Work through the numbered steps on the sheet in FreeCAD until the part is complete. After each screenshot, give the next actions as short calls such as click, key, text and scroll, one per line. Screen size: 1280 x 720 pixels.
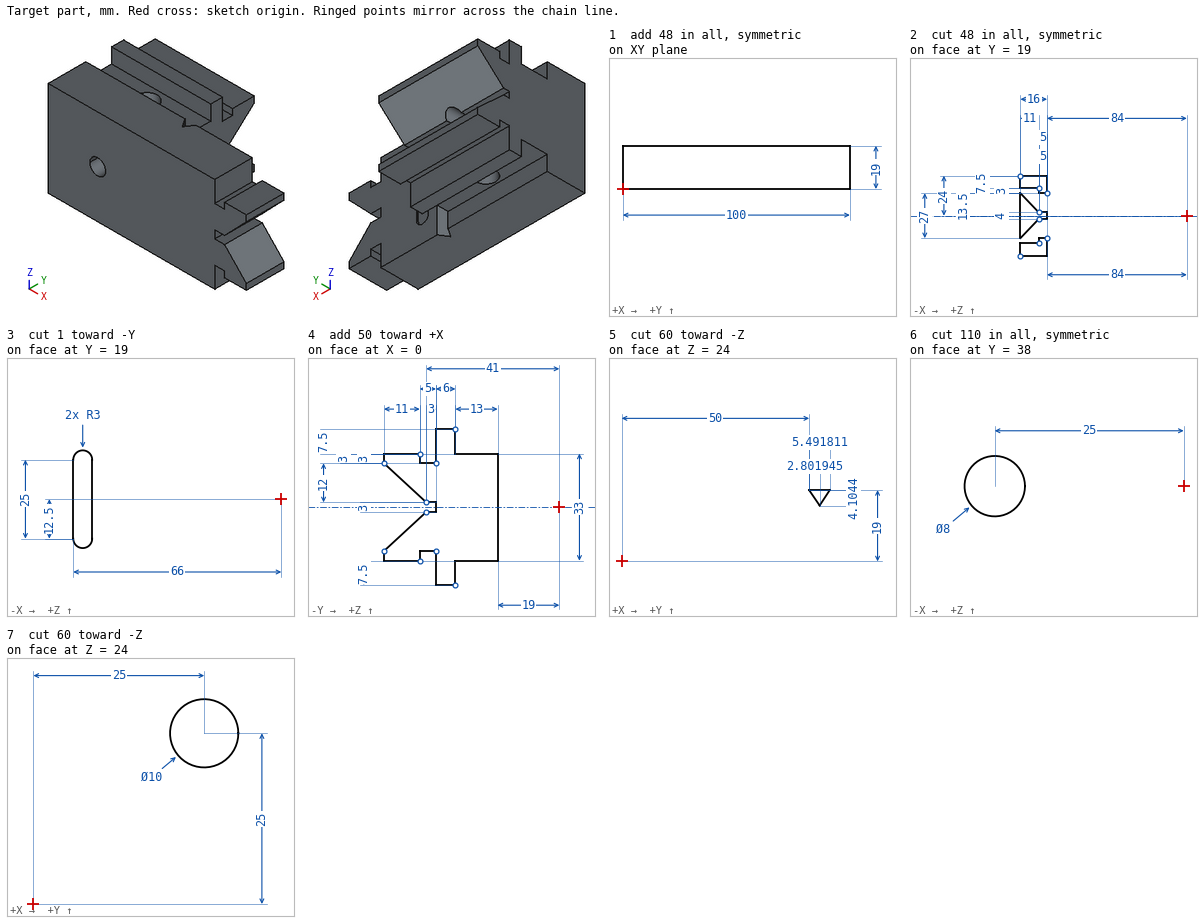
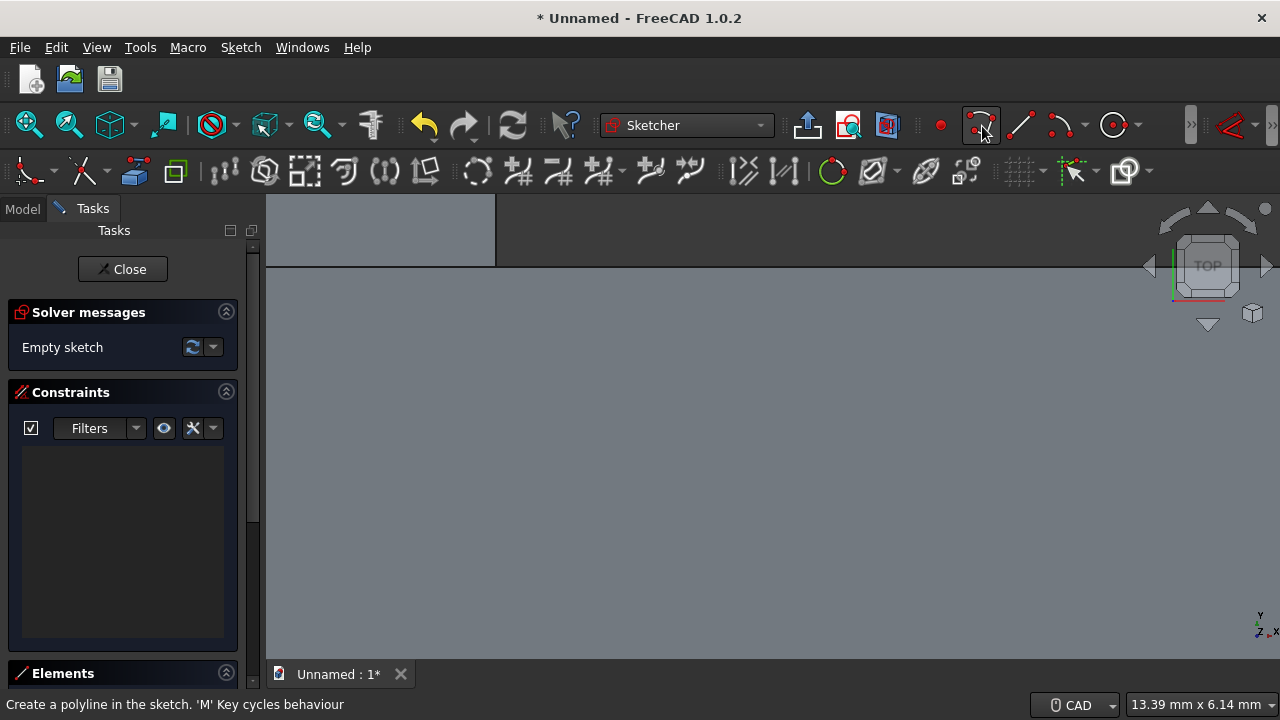
click(496, 267)
click(708, 578)
click(912, 267)
click(496, 268)
key(Escape)
key(Escape)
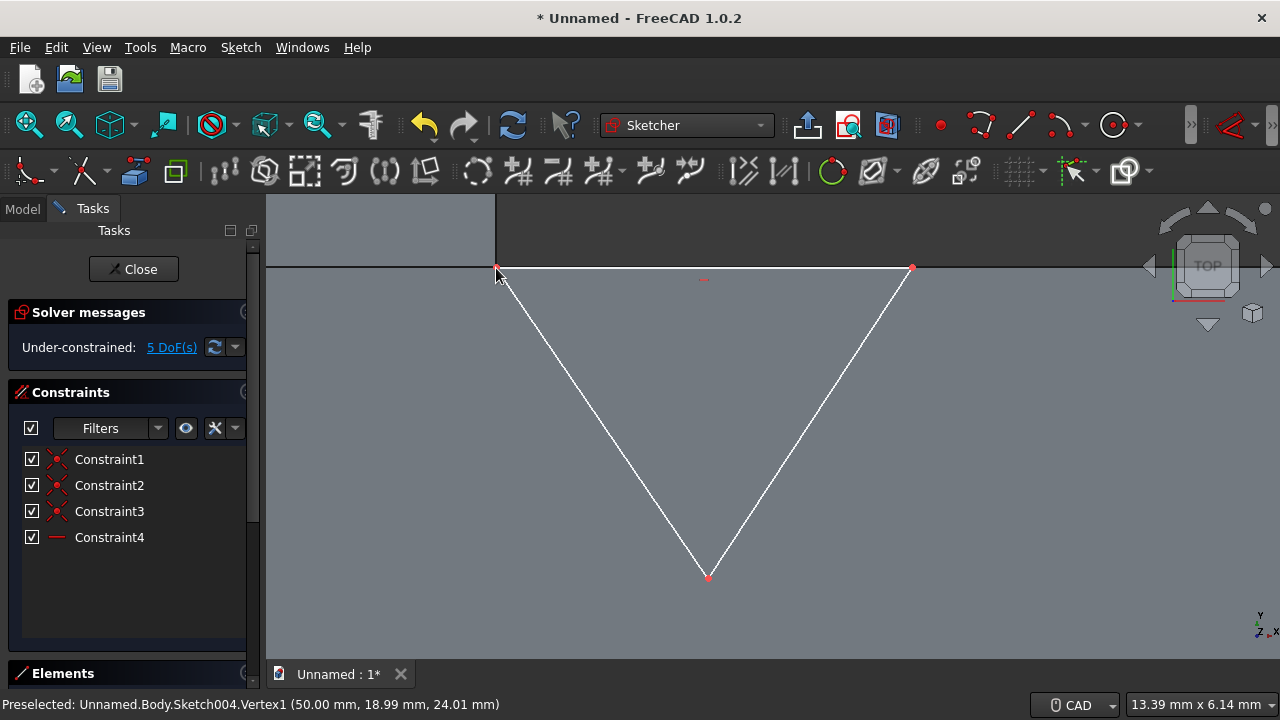
click(1230, 126)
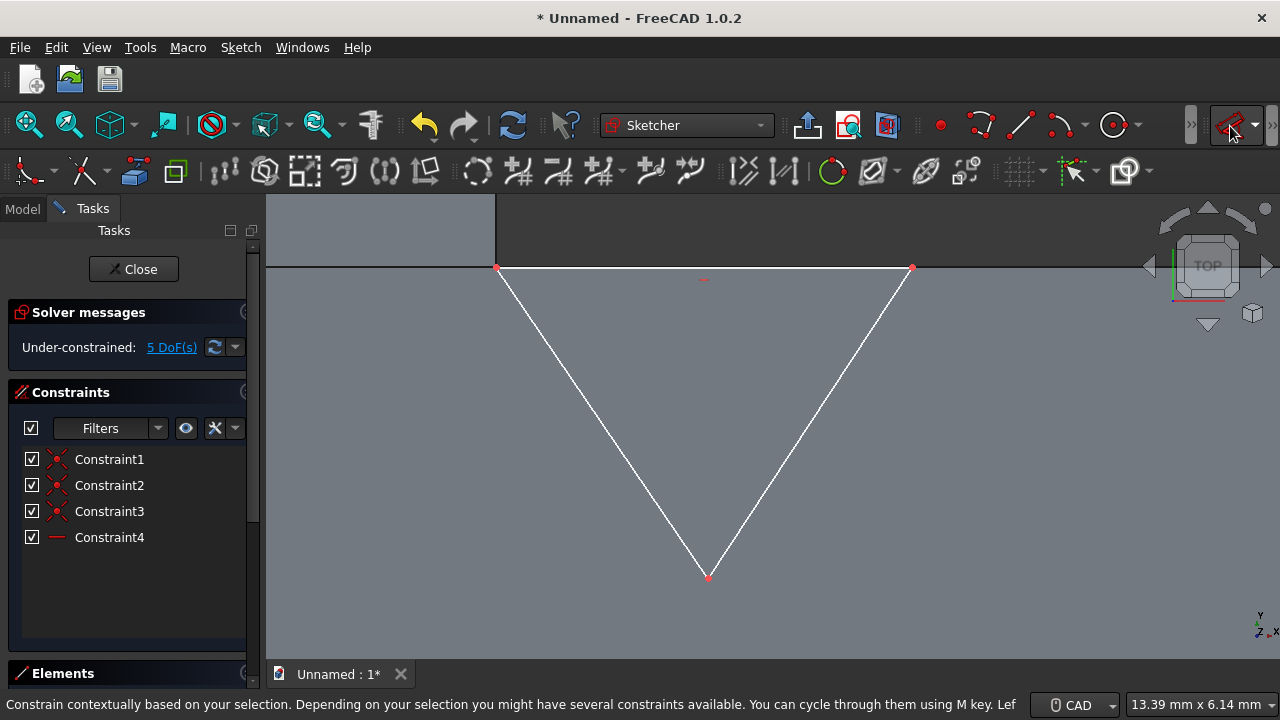
click(496, 268)
click(395, 234)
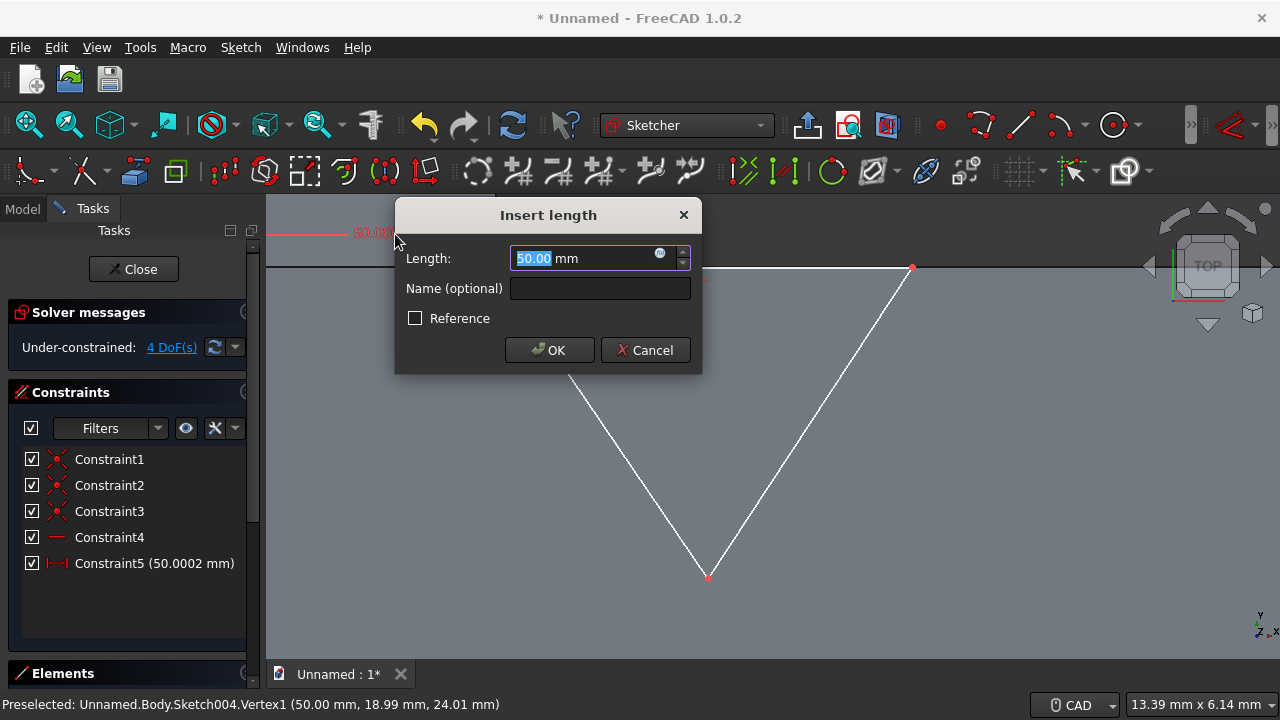
text(50)
key(Return)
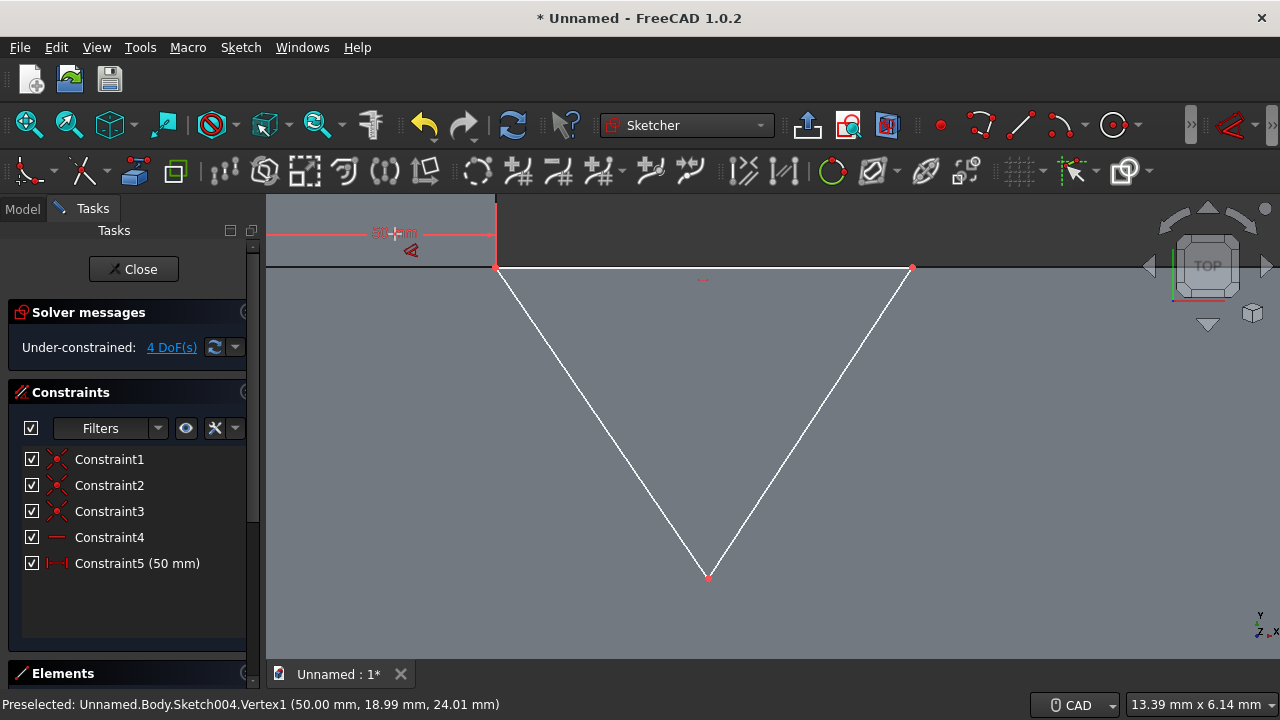
click(496, 268)
click(530, 450)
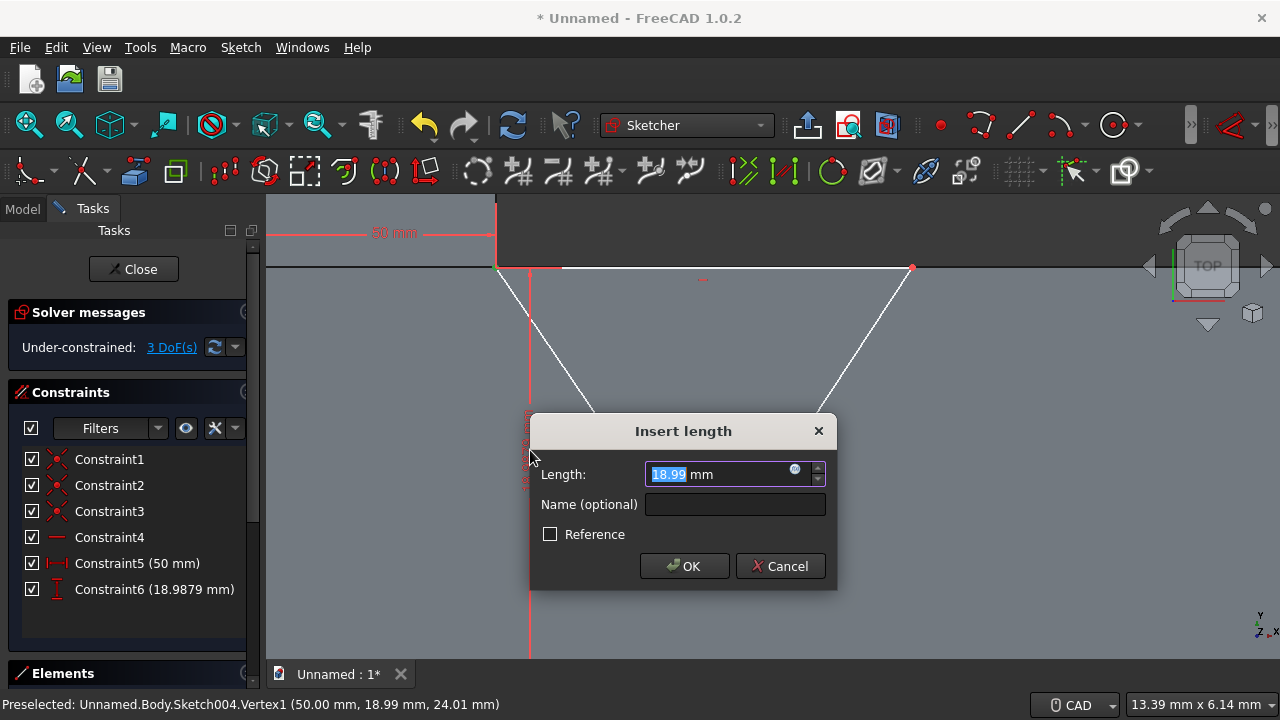
text(19)
key(Return)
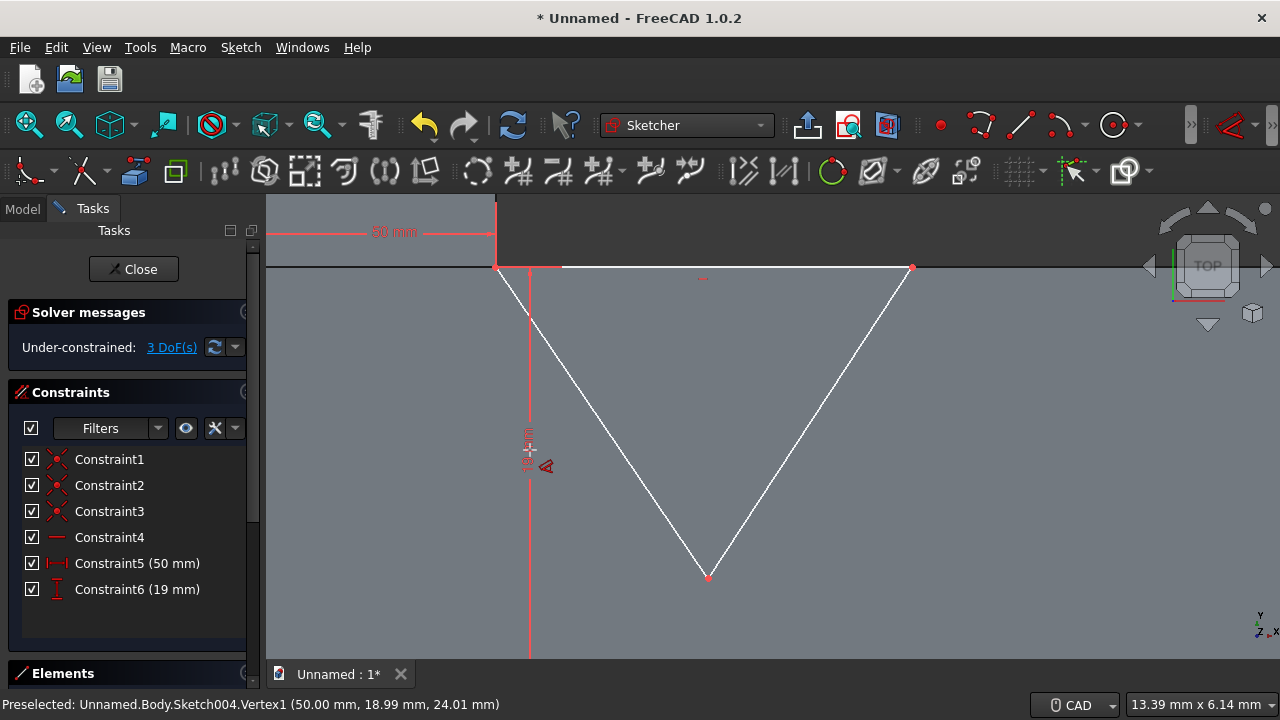
click(560, 361)
click(462, 423)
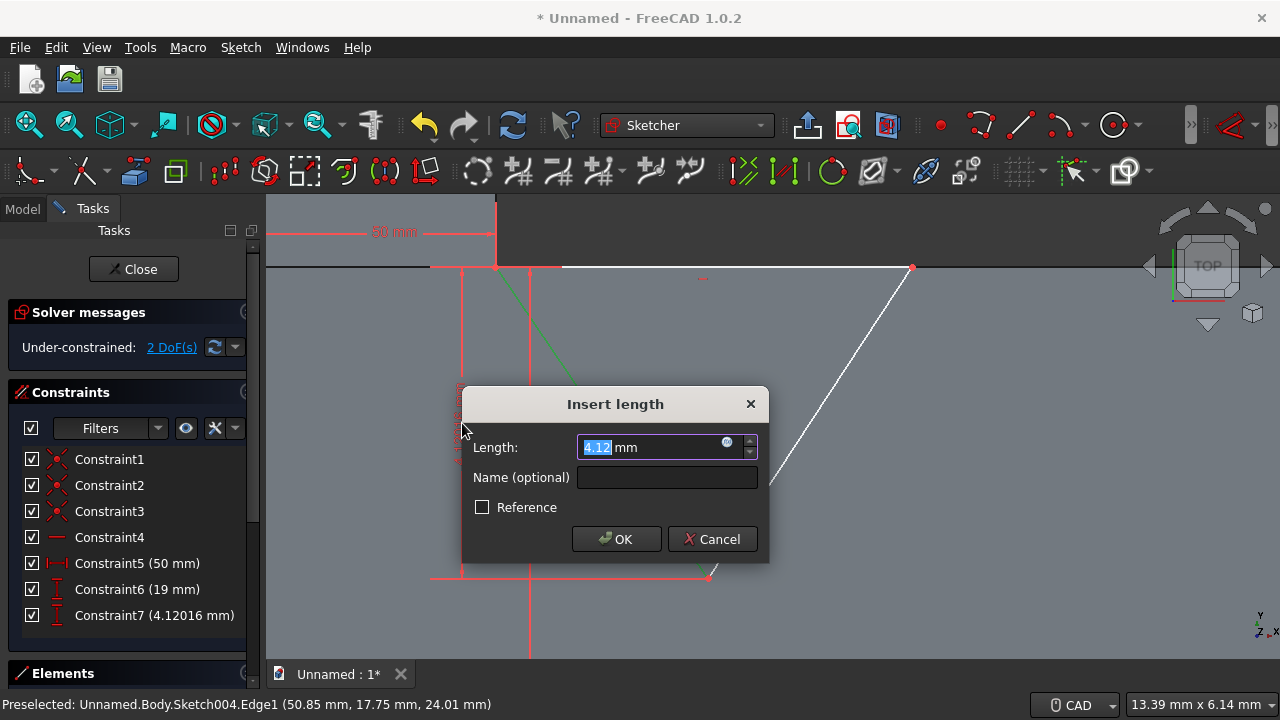
text(4.1044)
key(Return)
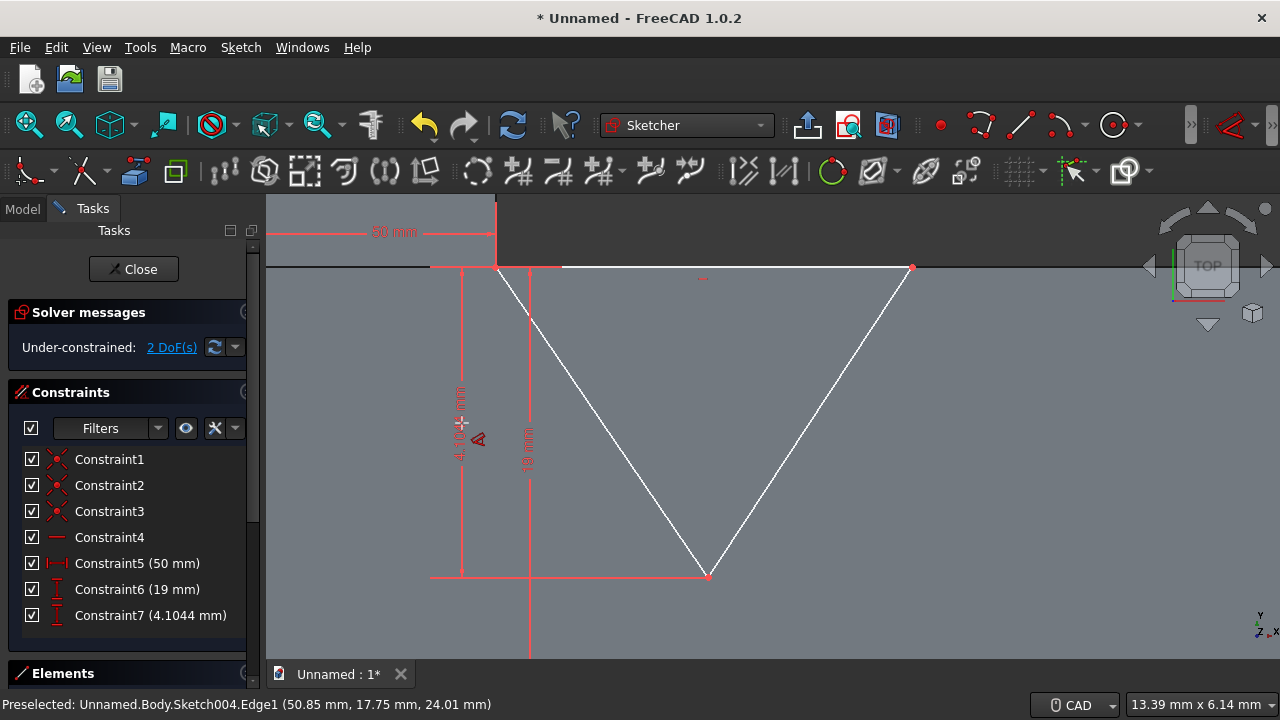
click(787, 267)
click(704, 233)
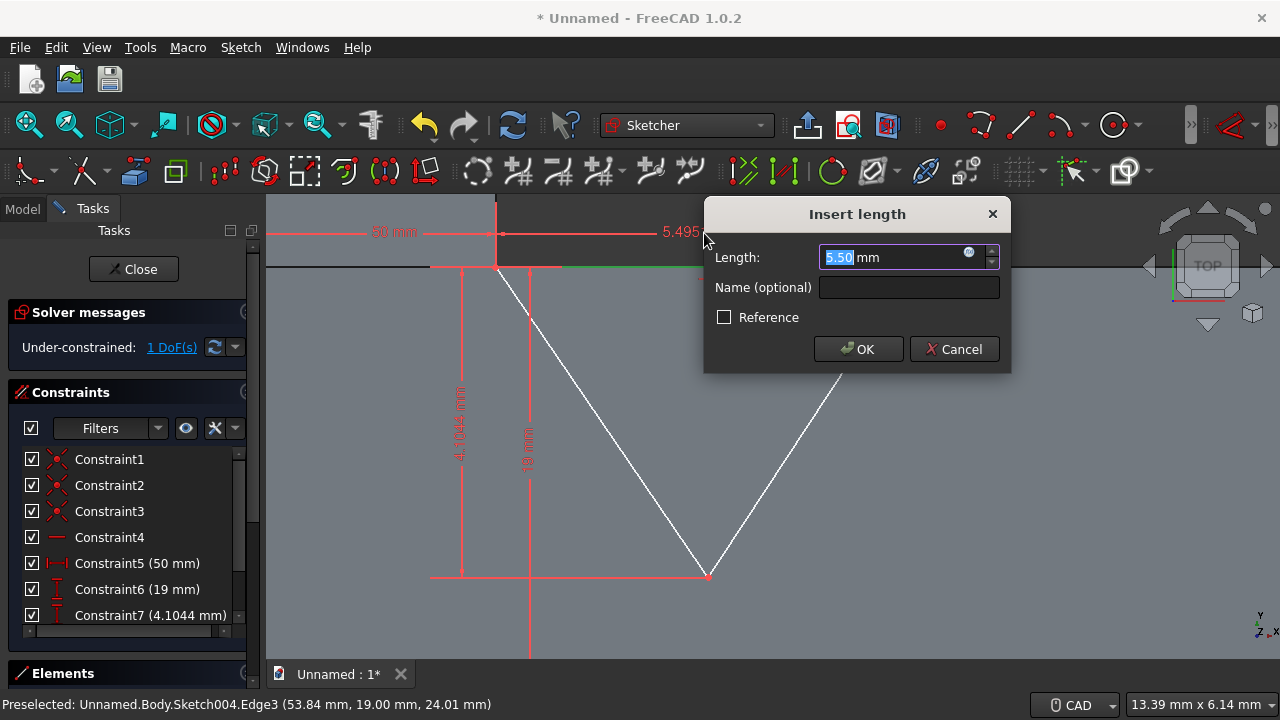
text(5.491811)
key(Return)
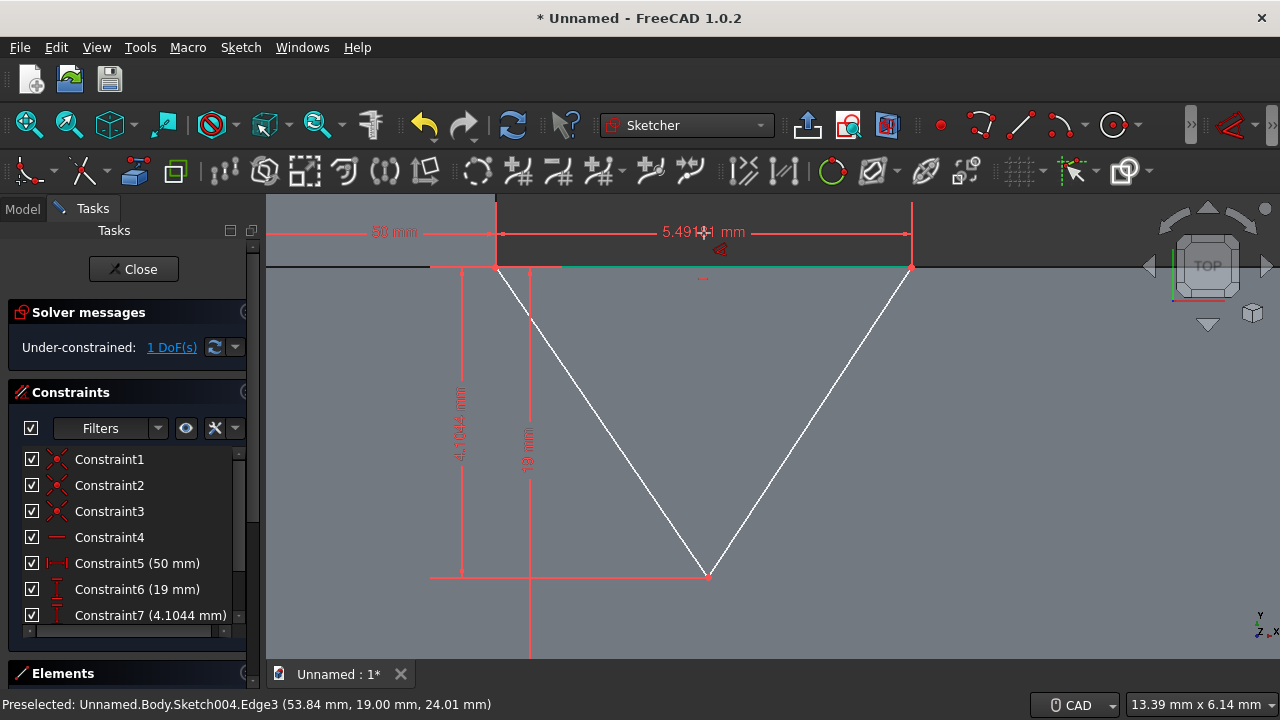
click(560, 360)
click(602, 233)